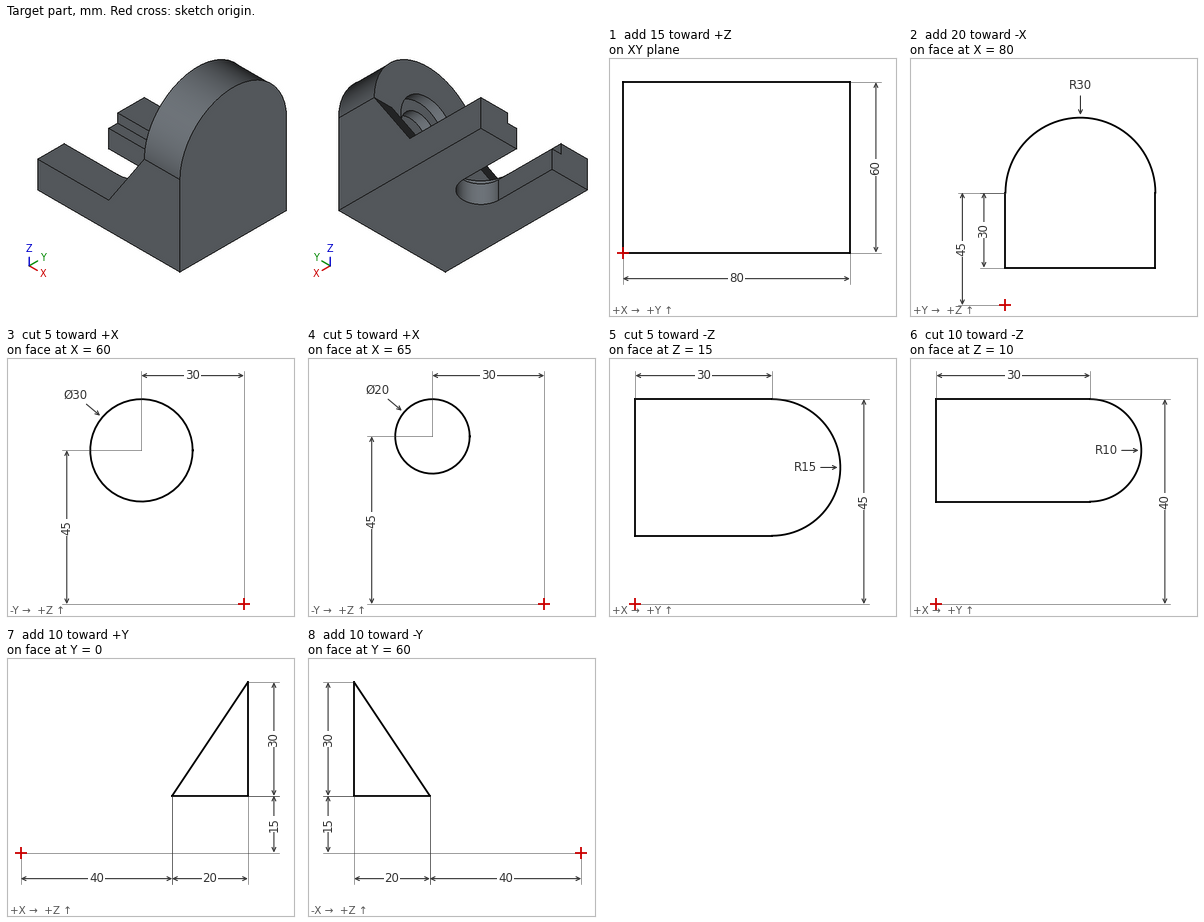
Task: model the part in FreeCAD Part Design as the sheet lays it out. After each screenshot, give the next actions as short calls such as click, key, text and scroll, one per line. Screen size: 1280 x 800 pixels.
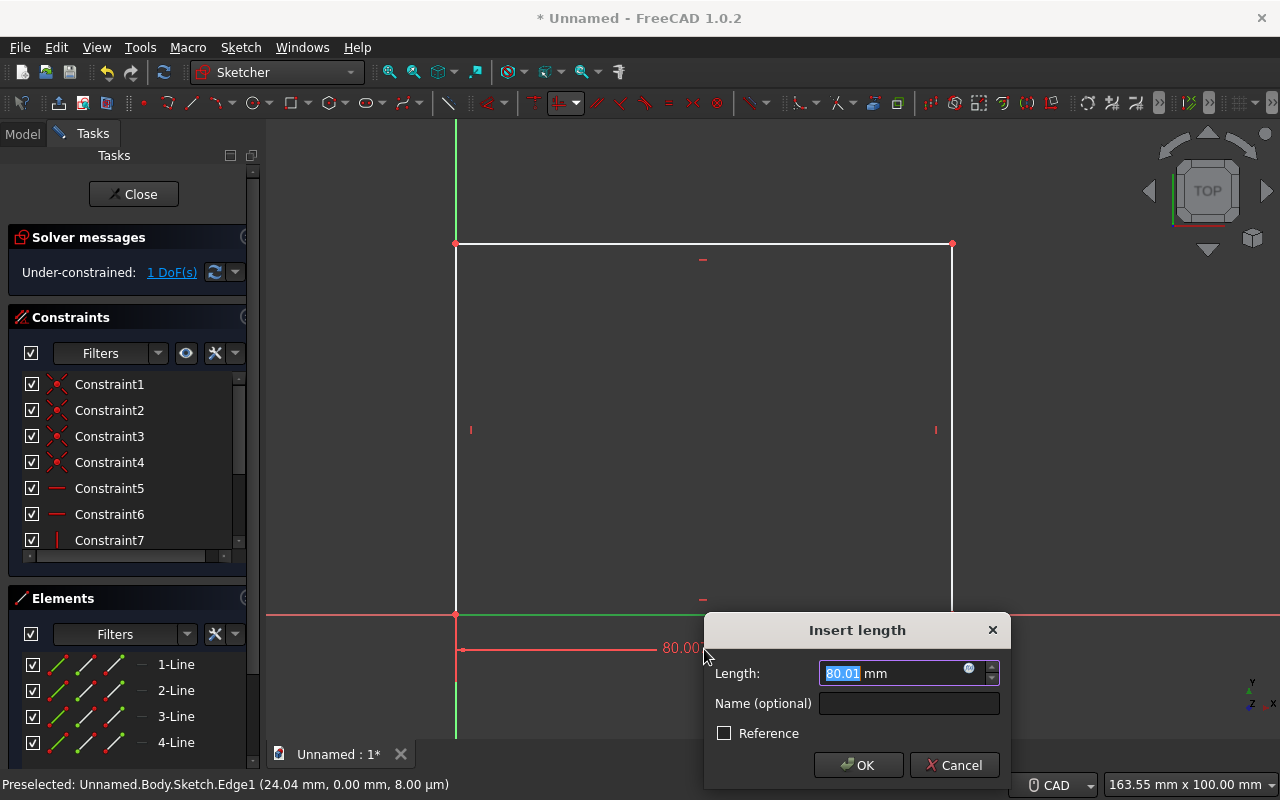
text(80)
key(Return)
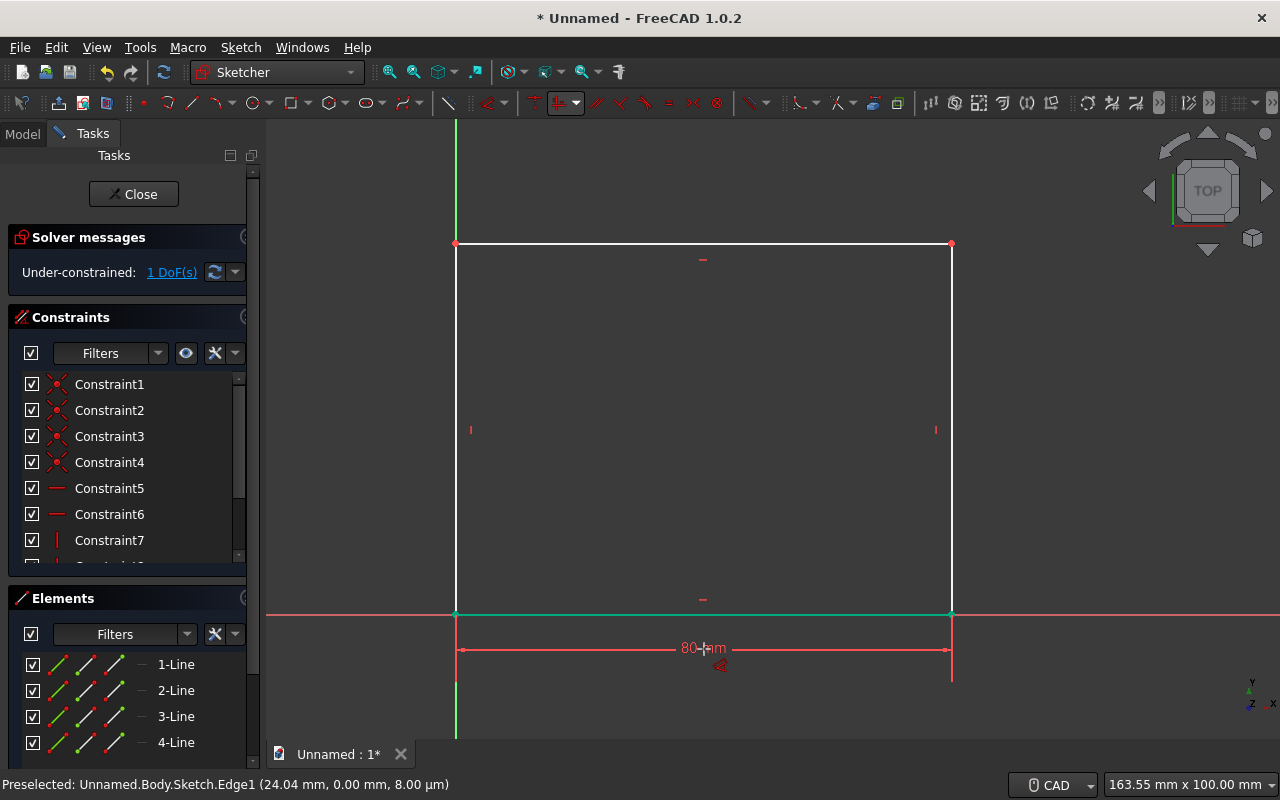
click(952, 504)
click(986, 429)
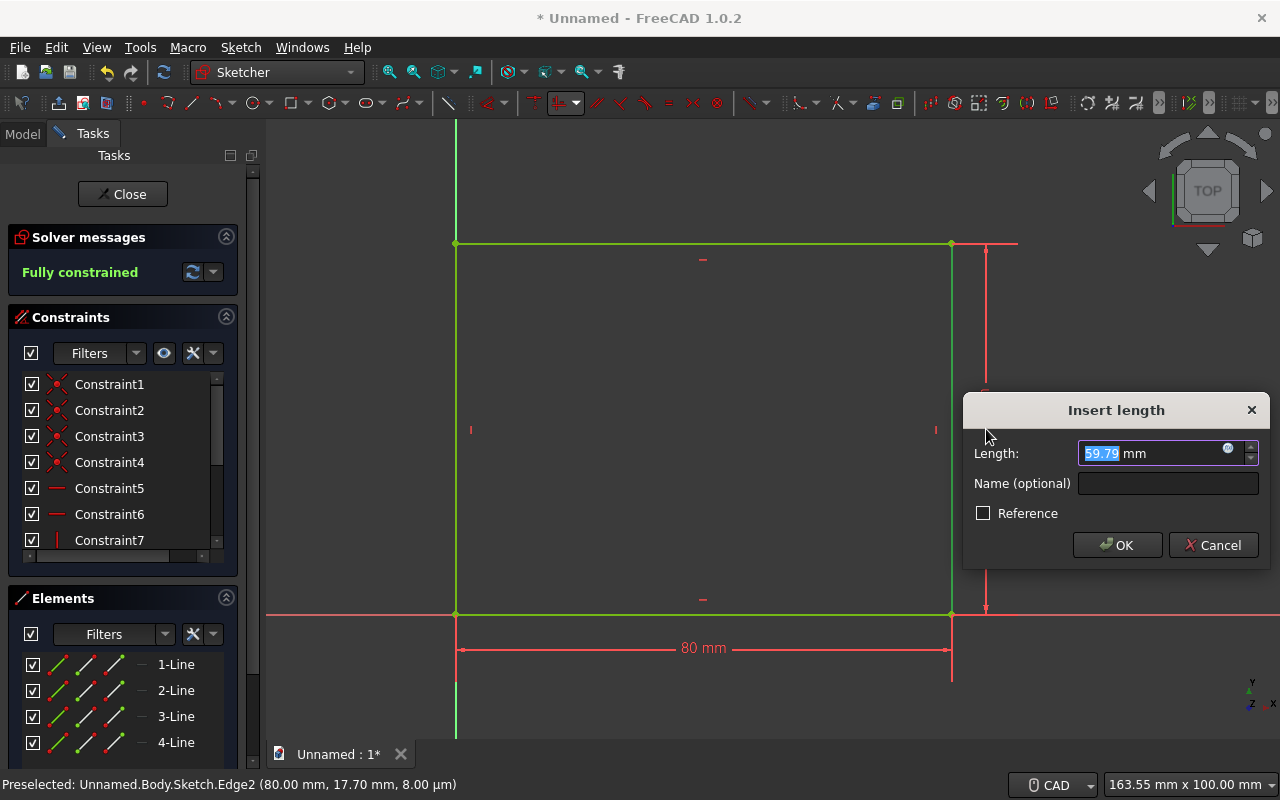
text(60)
key(Return)
key(Escape)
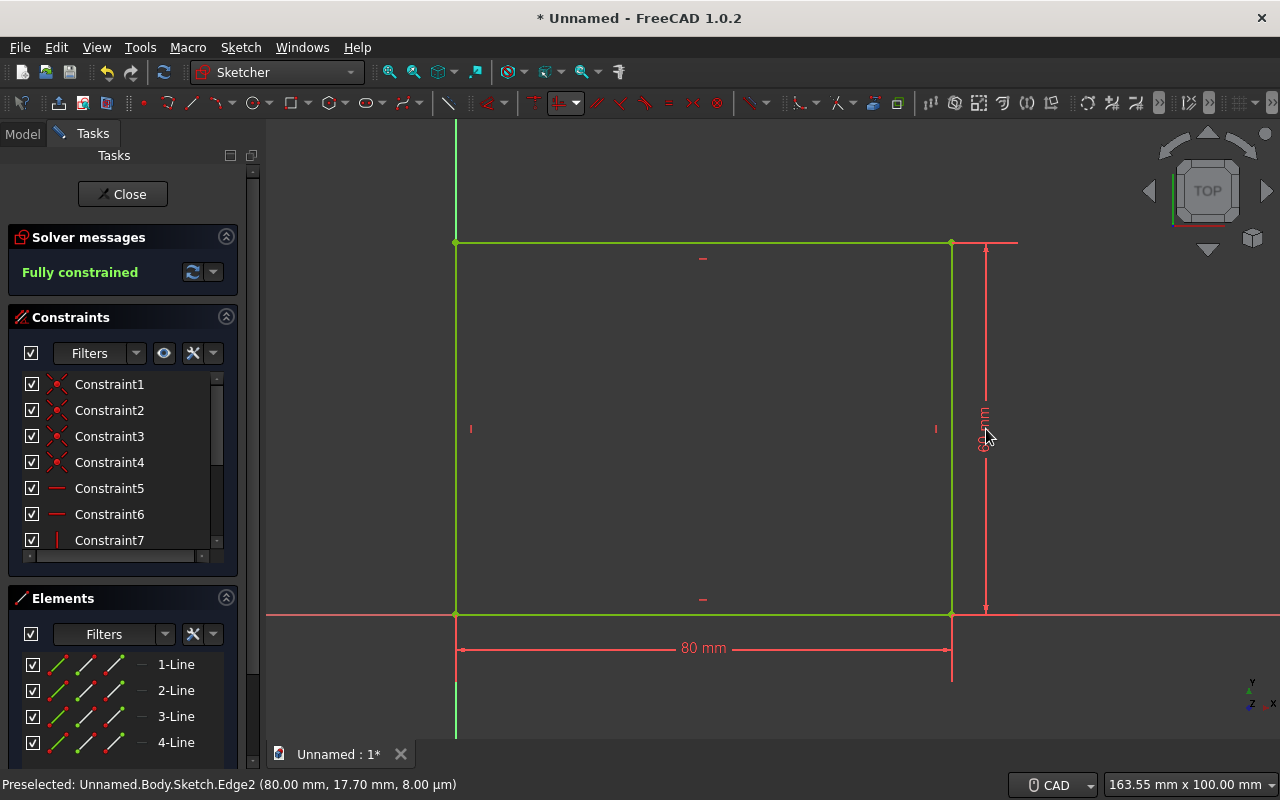
click(123, 194)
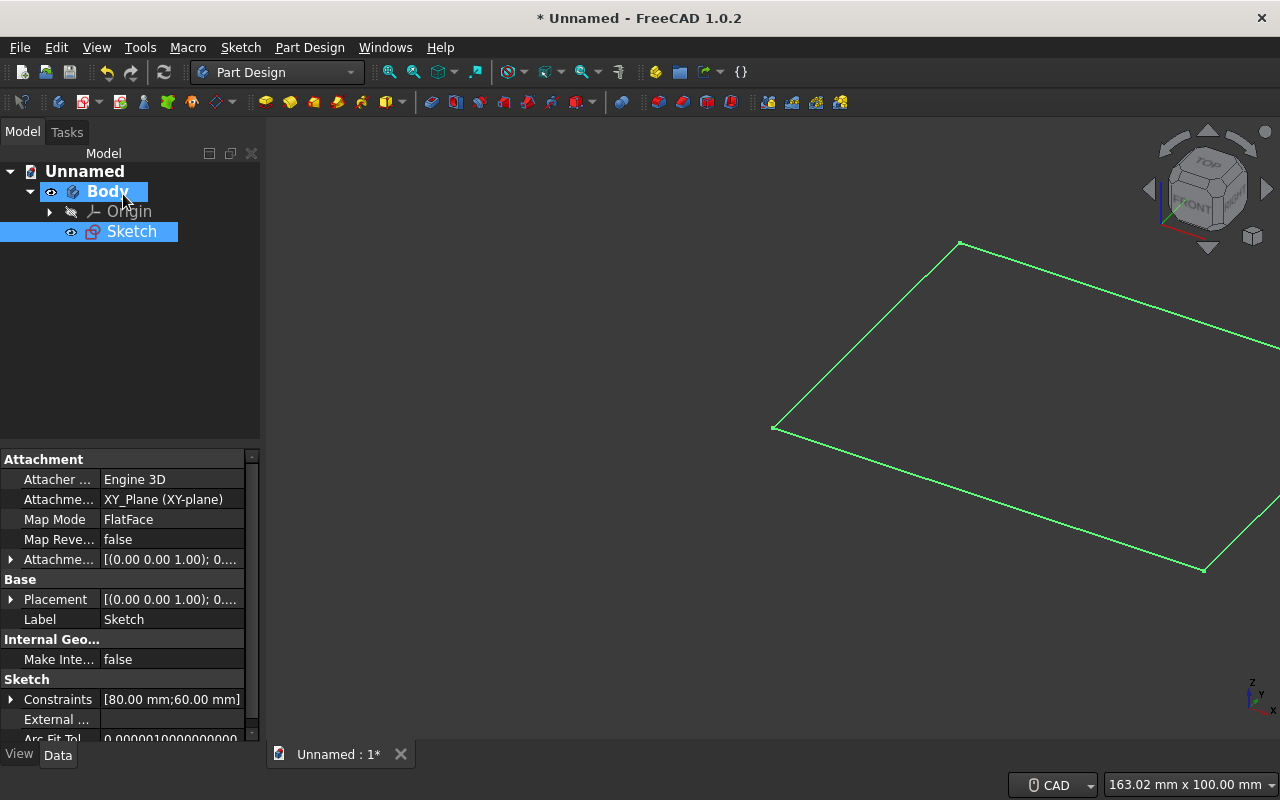
click(266, 102)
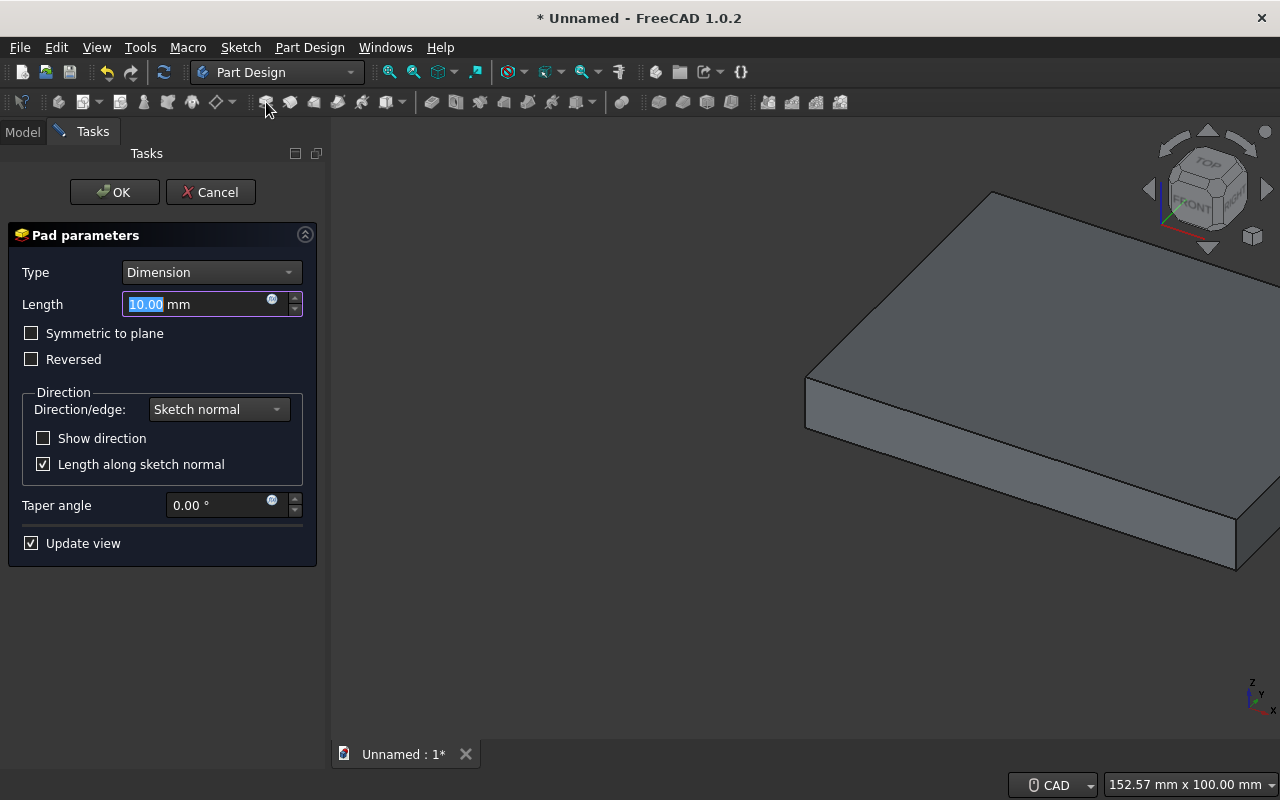
text(15)
key(Tab)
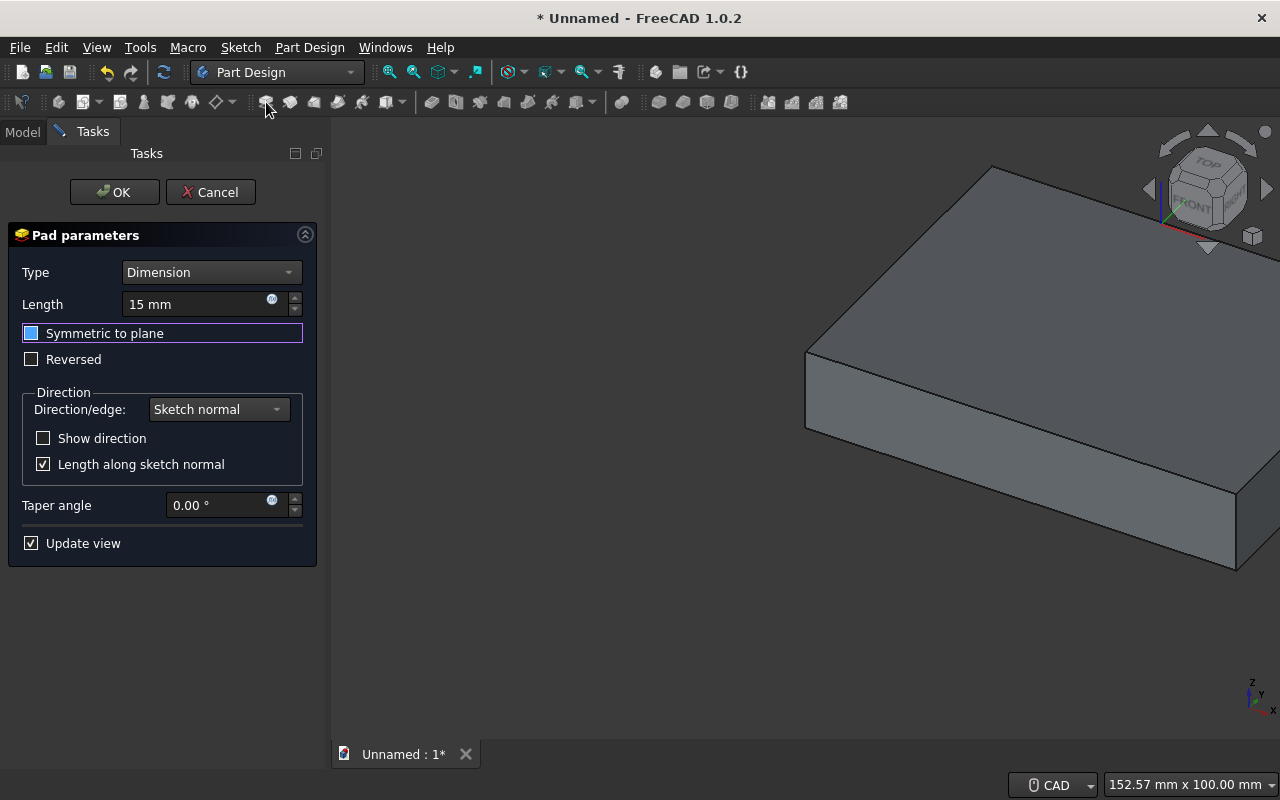
click(115, 192)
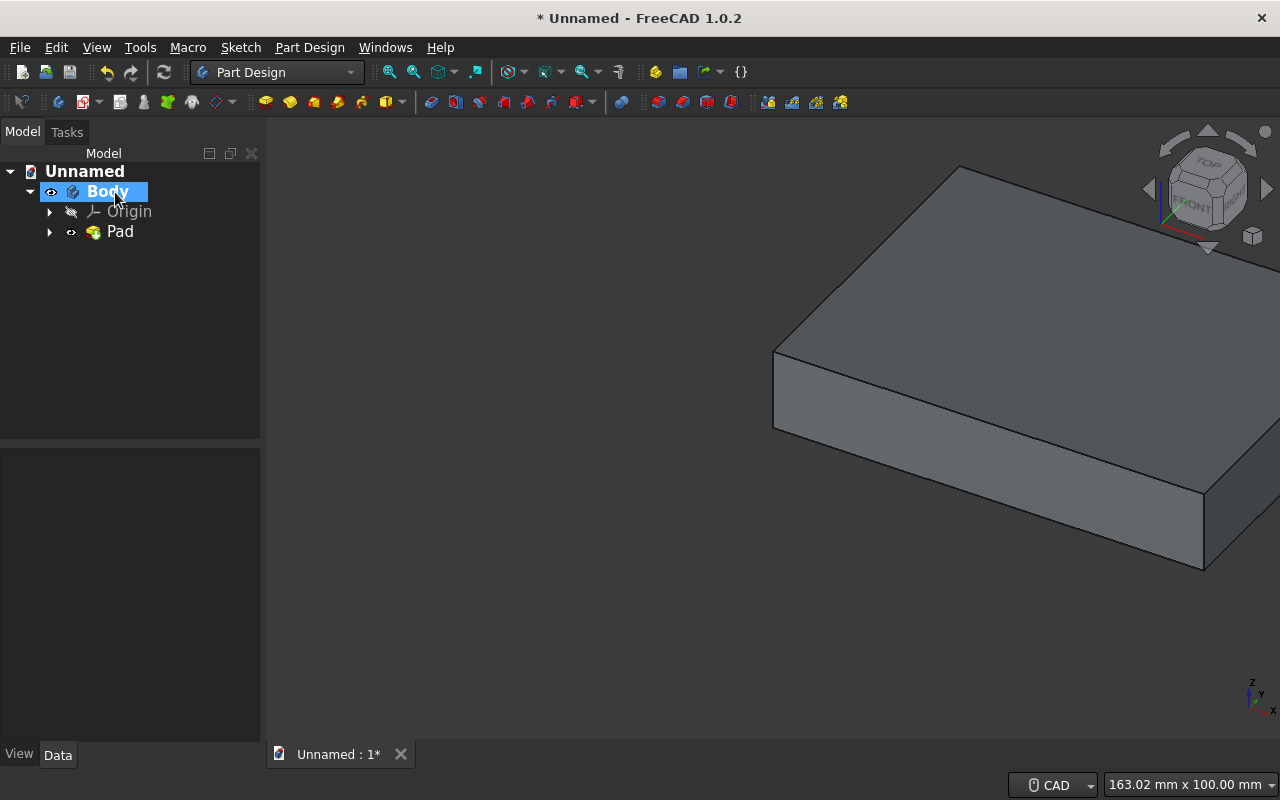
click(390, 72)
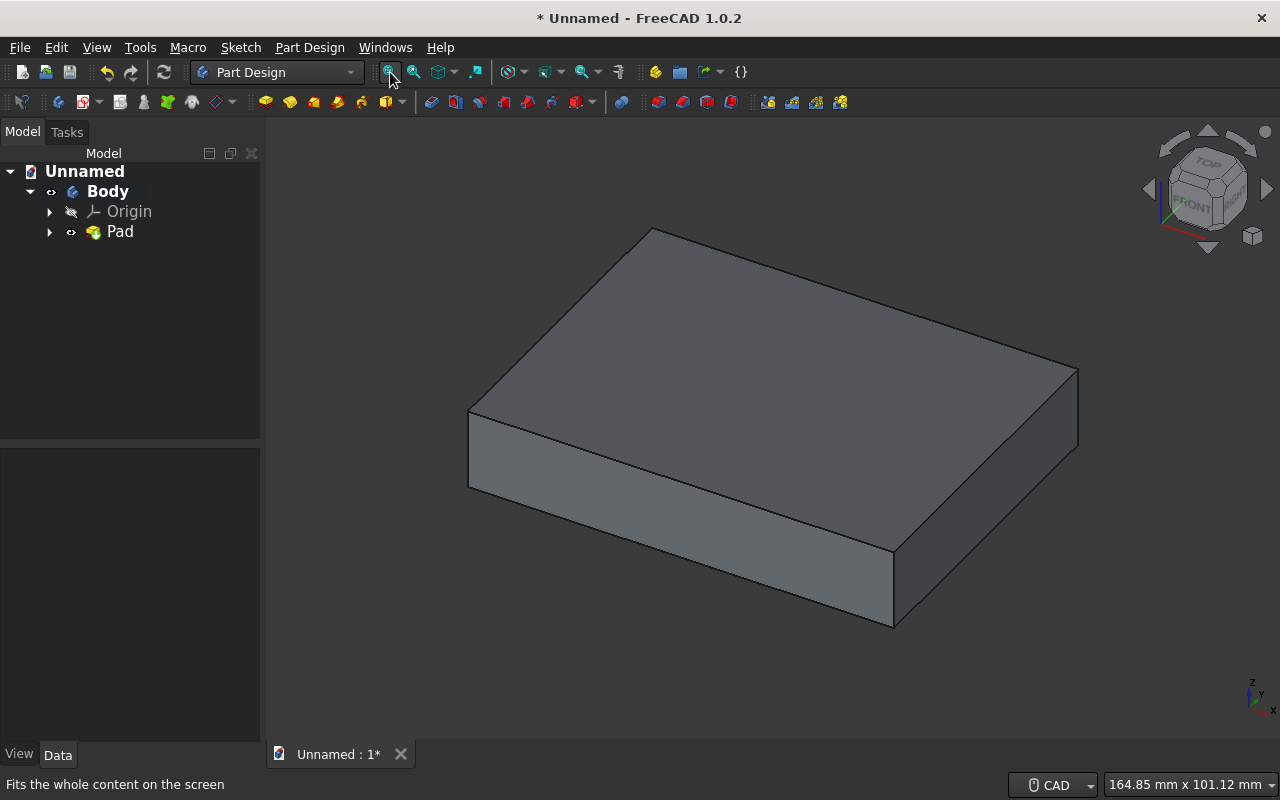
click(1039, 445)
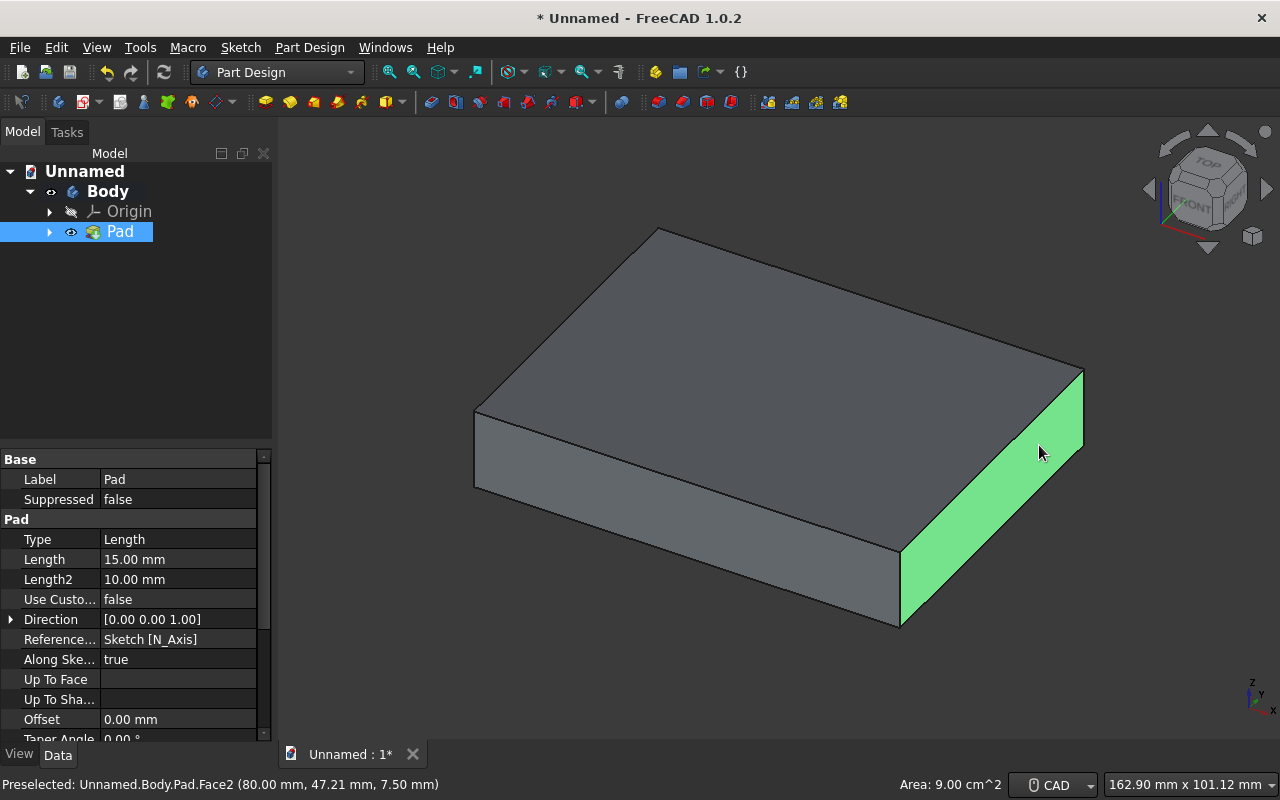
click(84, 102)